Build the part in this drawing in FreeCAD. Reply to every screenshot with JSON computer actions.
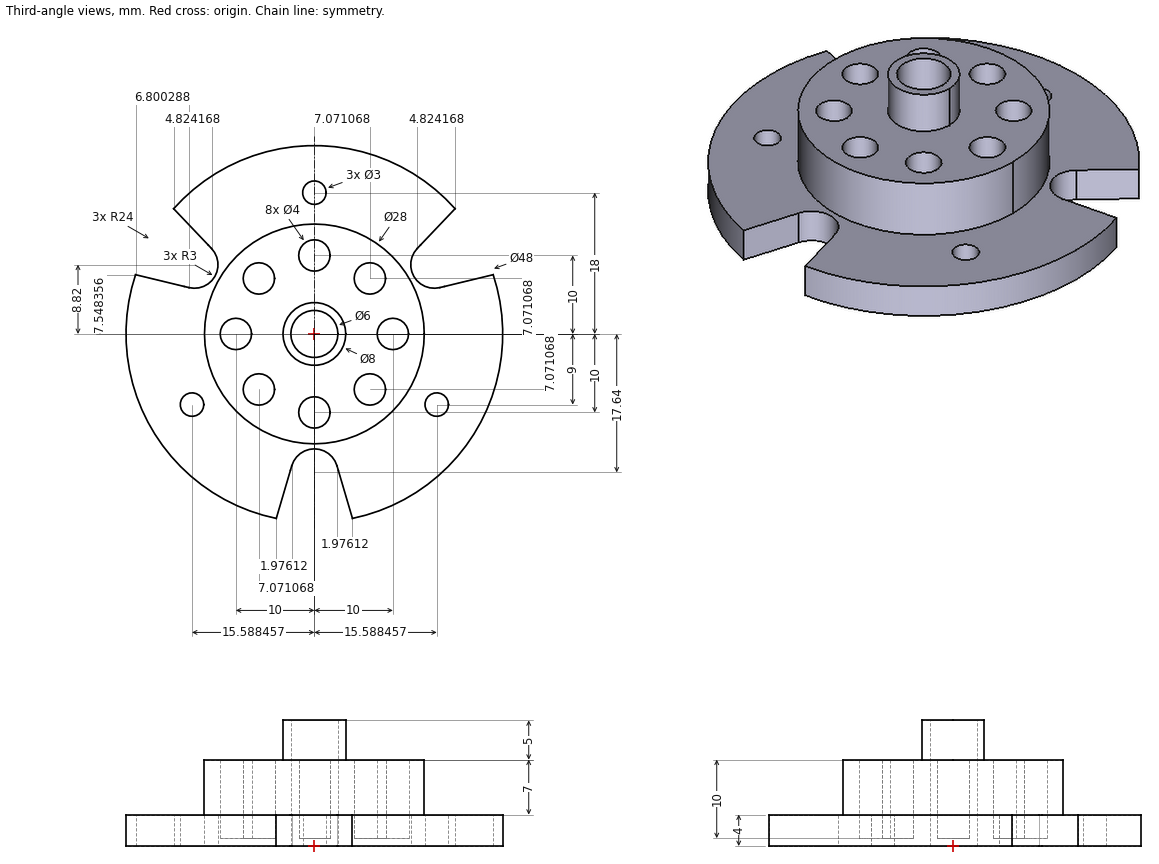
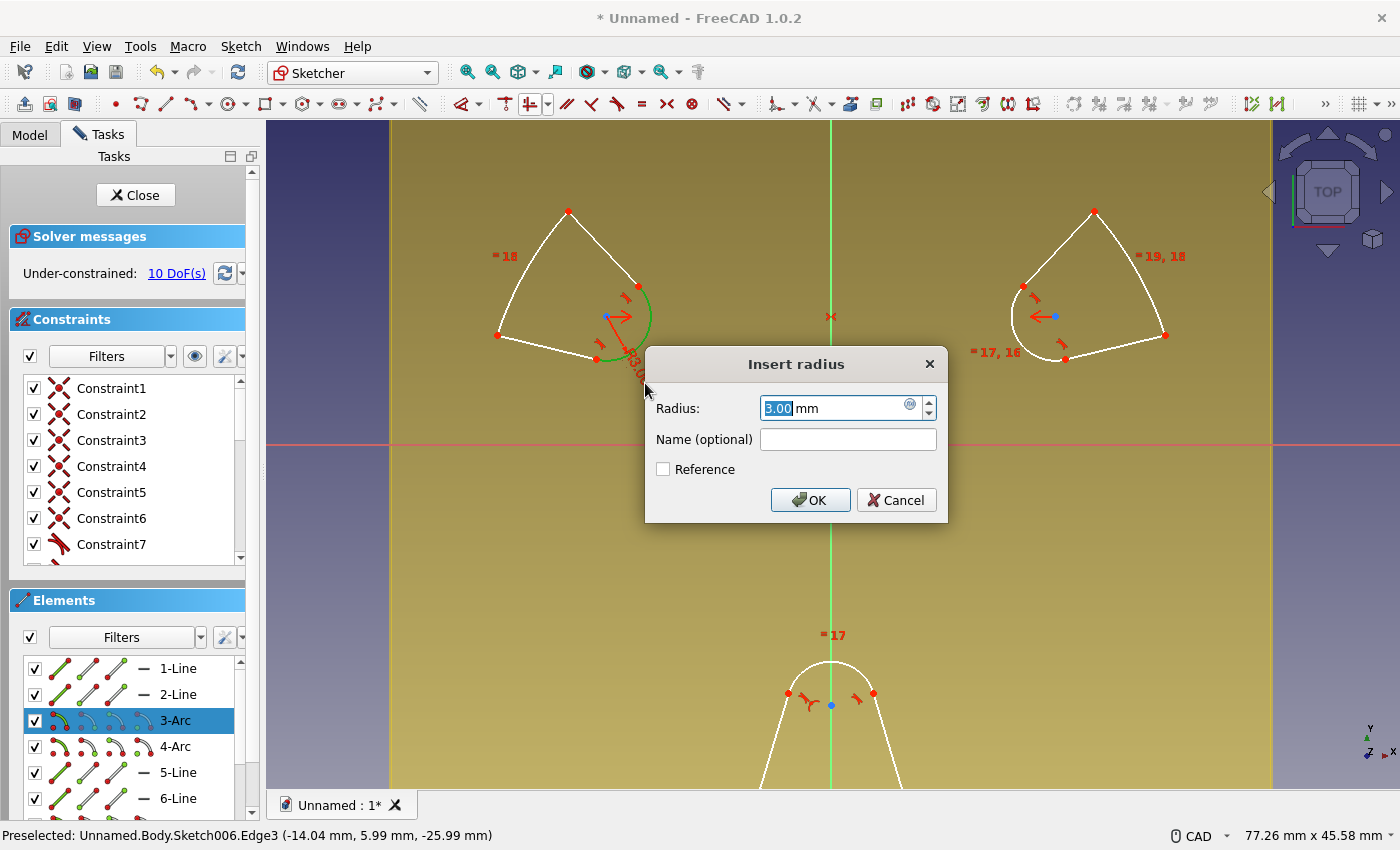
{"action": "type", "text": "3"}
{"action": "key", "text": "Return"}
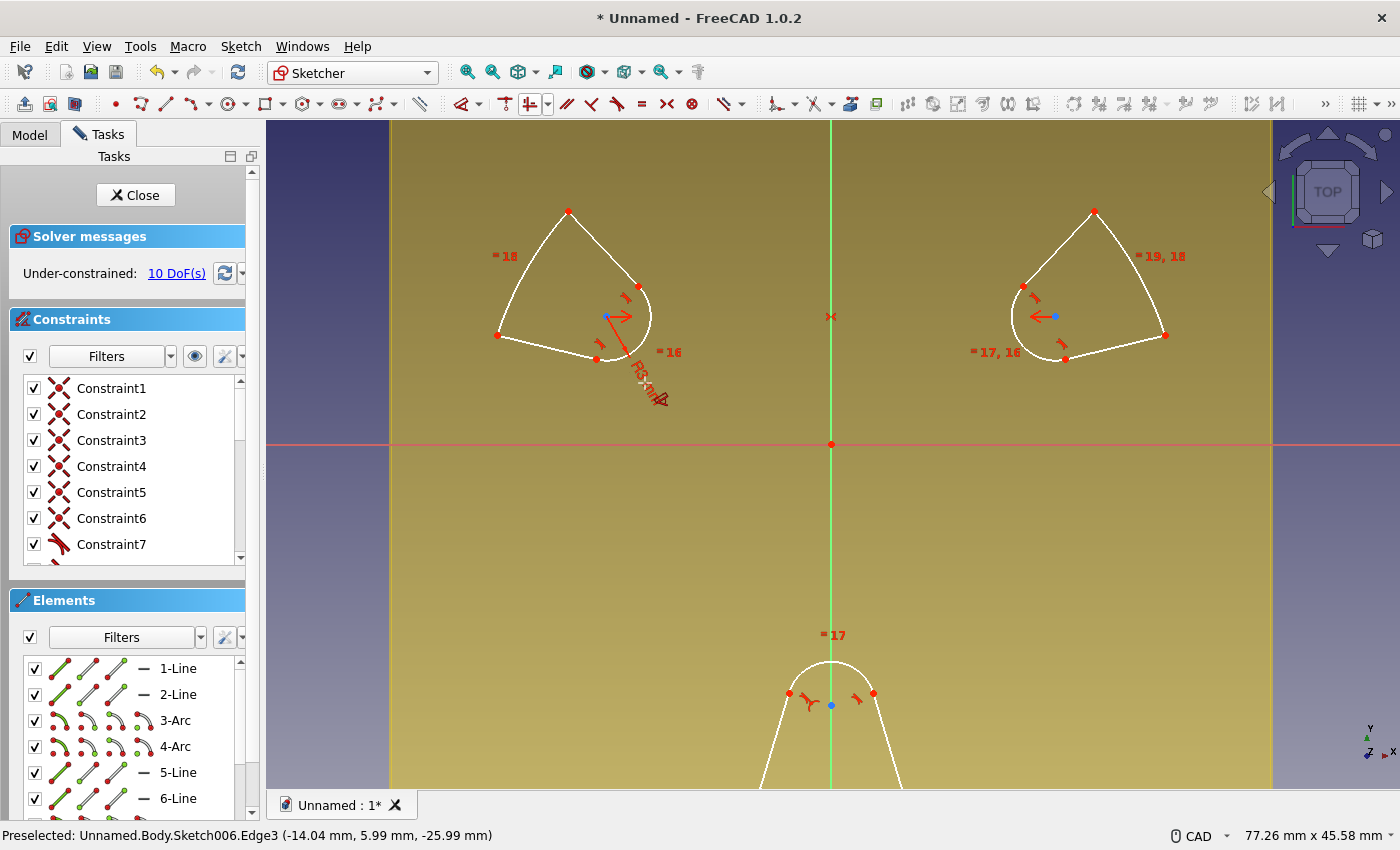
{"action": "left_click", "coordinate": [542, 246]}
{"action": "left_click", "coordinate": [516, 228]}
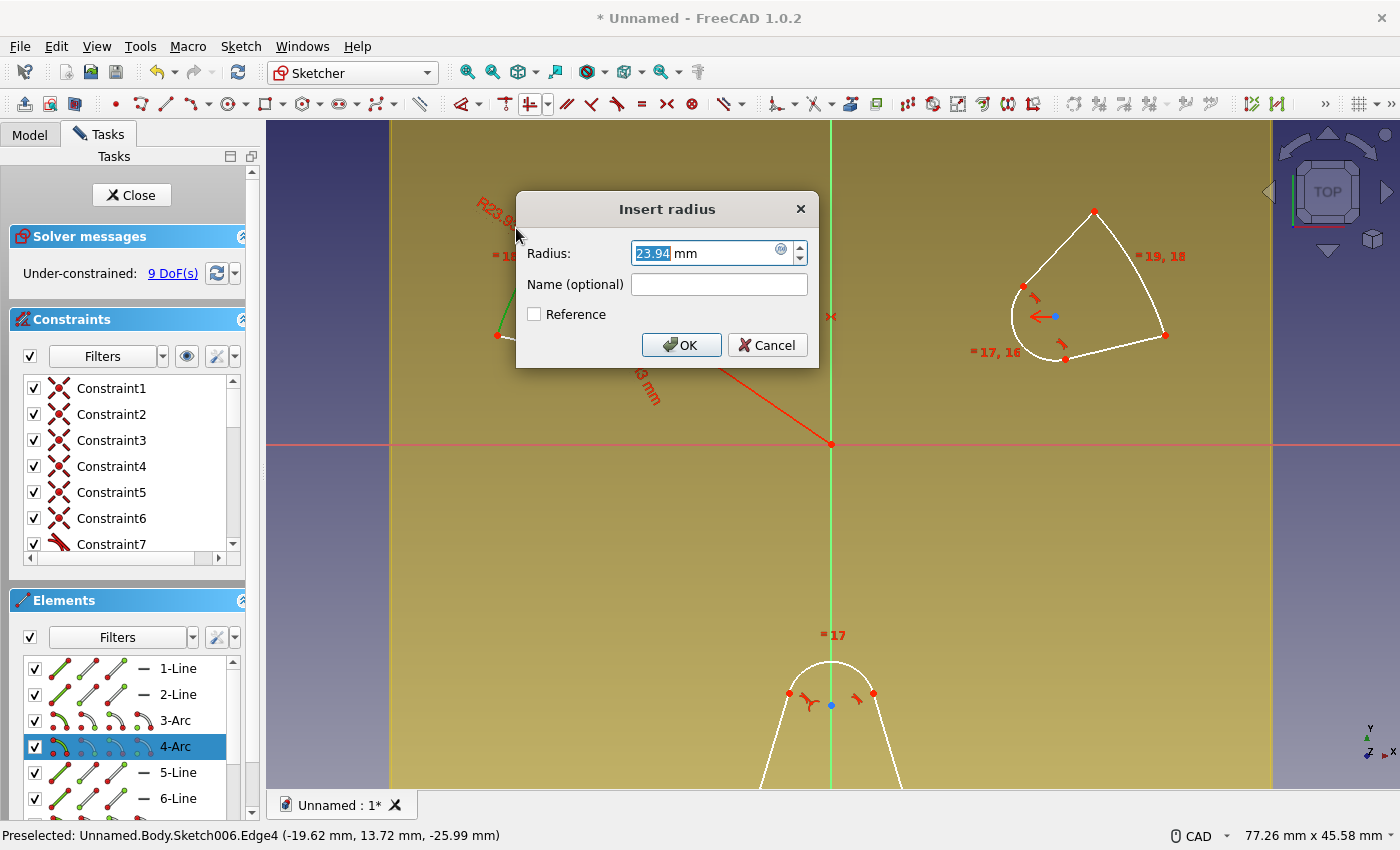
{"action": "type", "text": "24"}
{"action": "key", "text": "Return"}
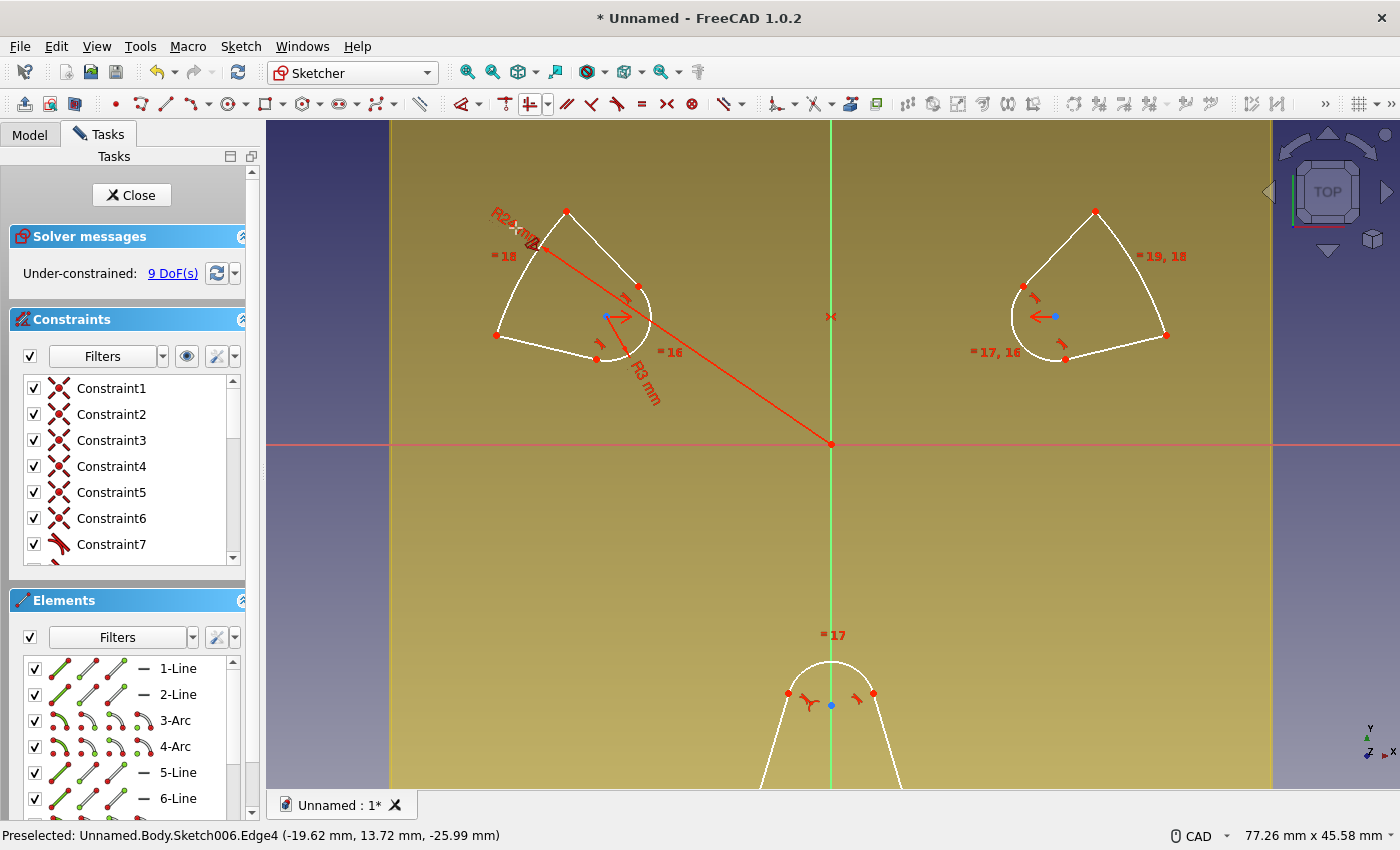
{"action": "left_click", "coordinate": [607, 317]}
{"action": "left_click", "coordinate": [573, 381]}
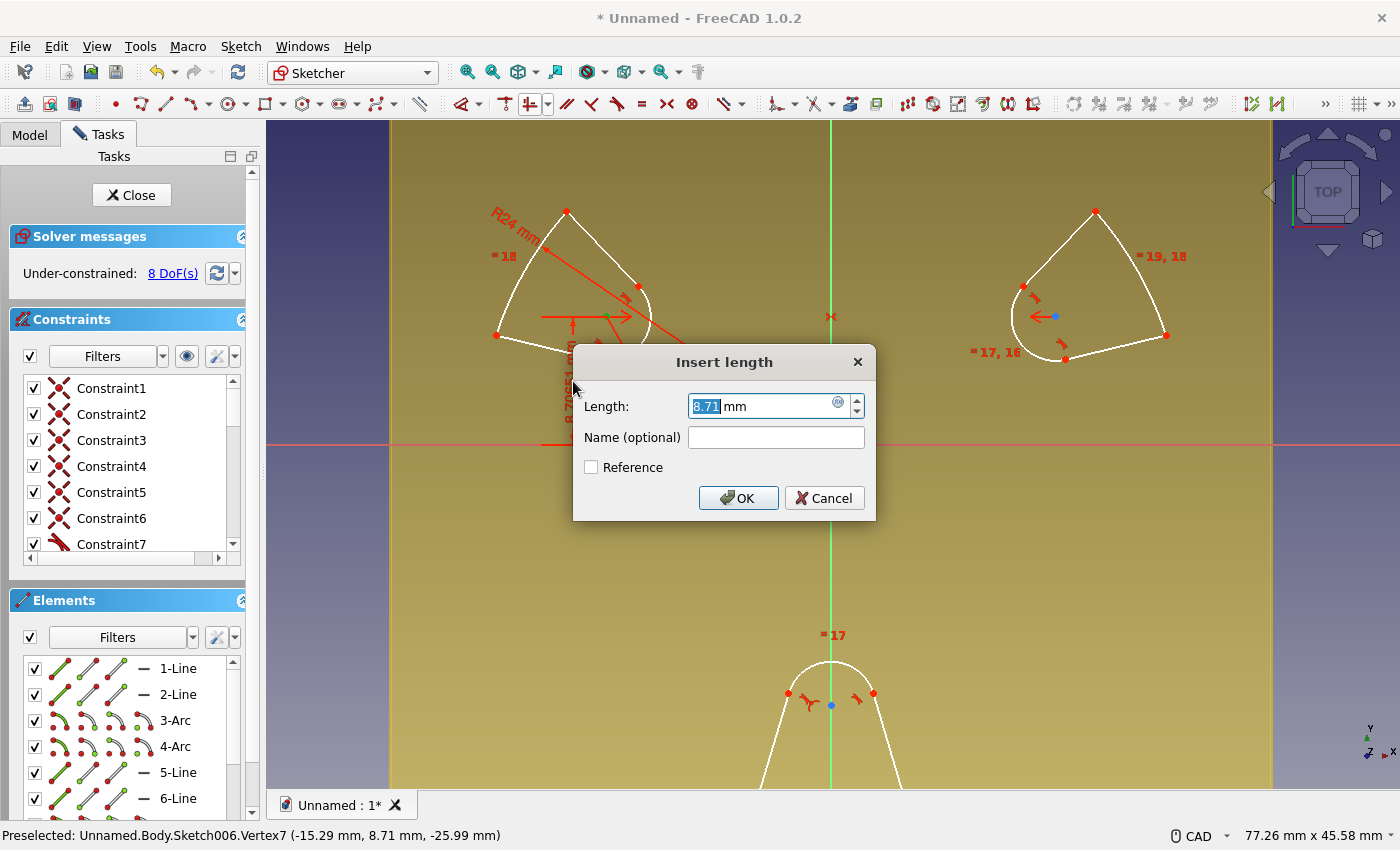
{"action": "type", "text": "8.82"}
{"action": "key", "text": "Return"}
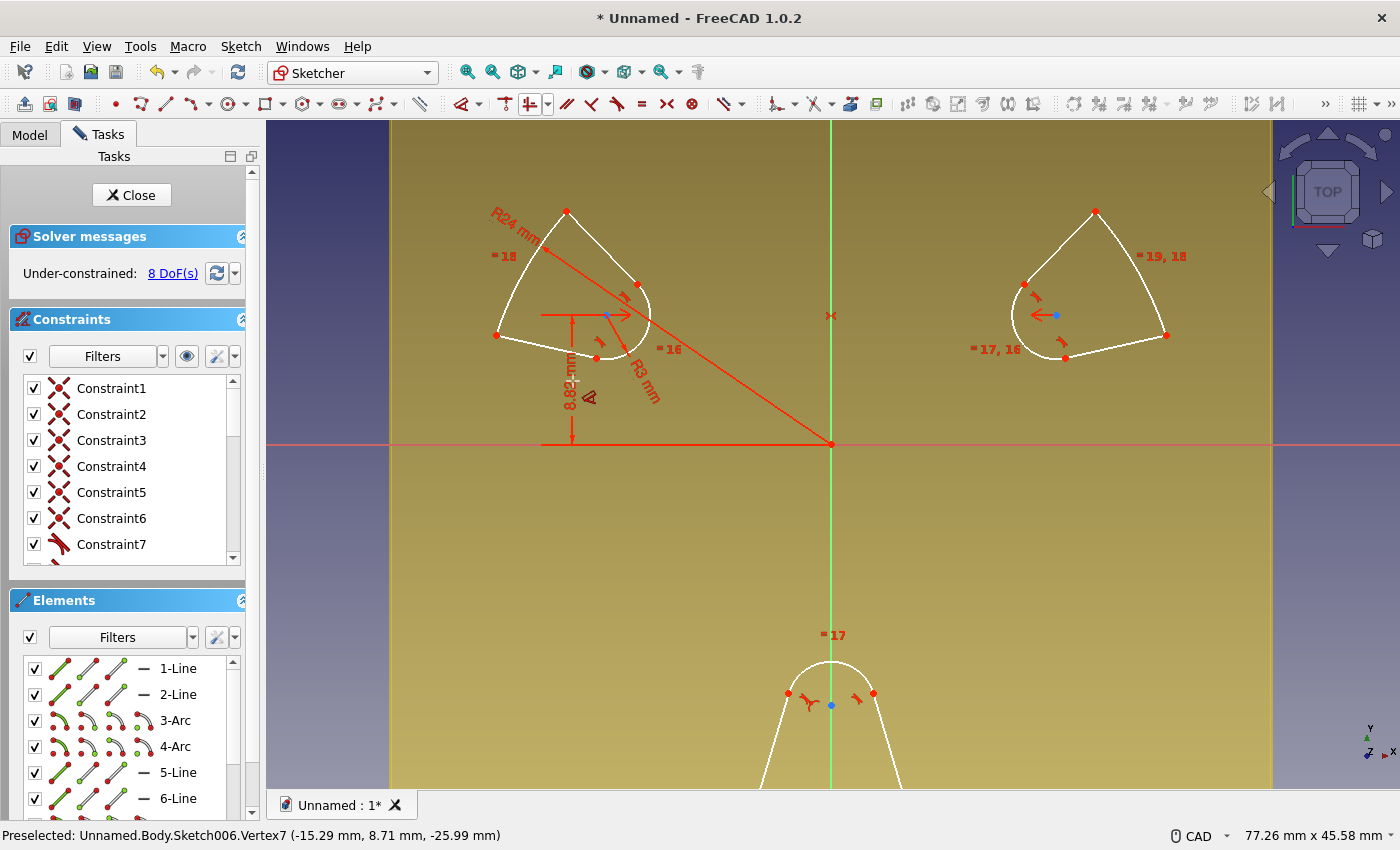
{"action": "left_click", "coordinate": [831, 706]}
{"action": "left_click", "coordinate": [865, 575]}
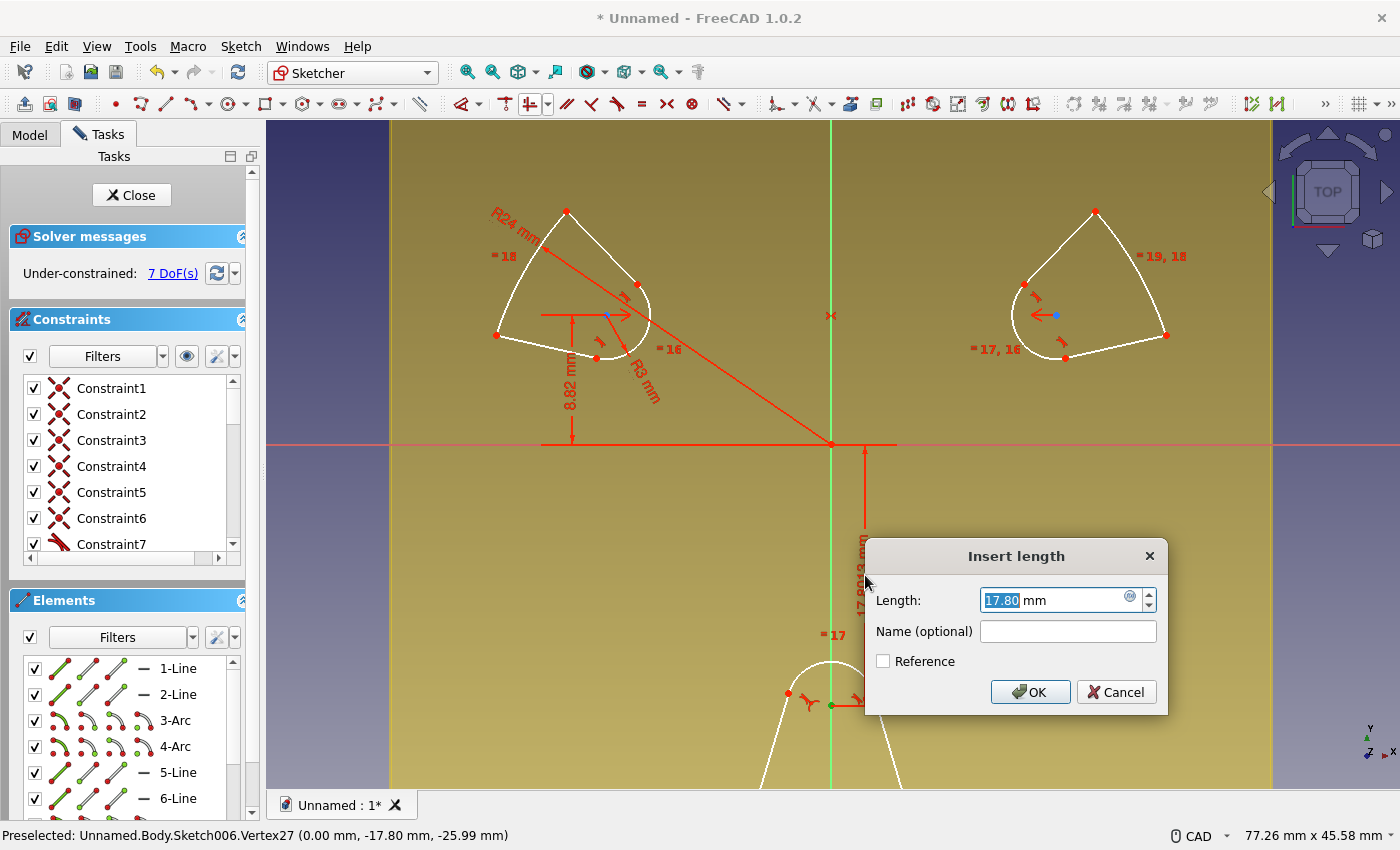
{"action": "type", "text": "17.64"}
{"action": "key", "text": "Return"}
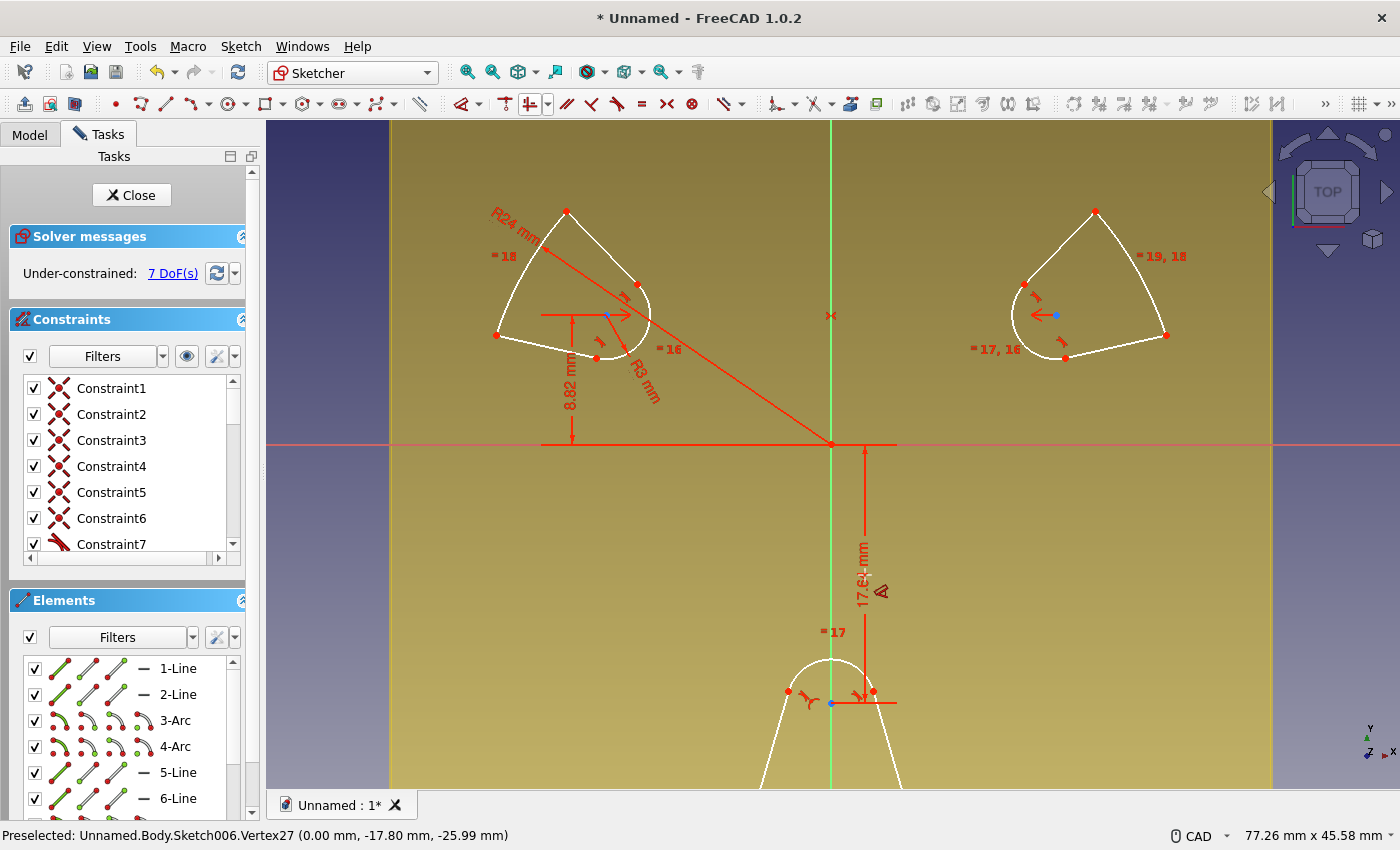
{"action": "scroll", "coordinate": [893, 760], "scroll_direction": "up", "scroll_amount": 2}